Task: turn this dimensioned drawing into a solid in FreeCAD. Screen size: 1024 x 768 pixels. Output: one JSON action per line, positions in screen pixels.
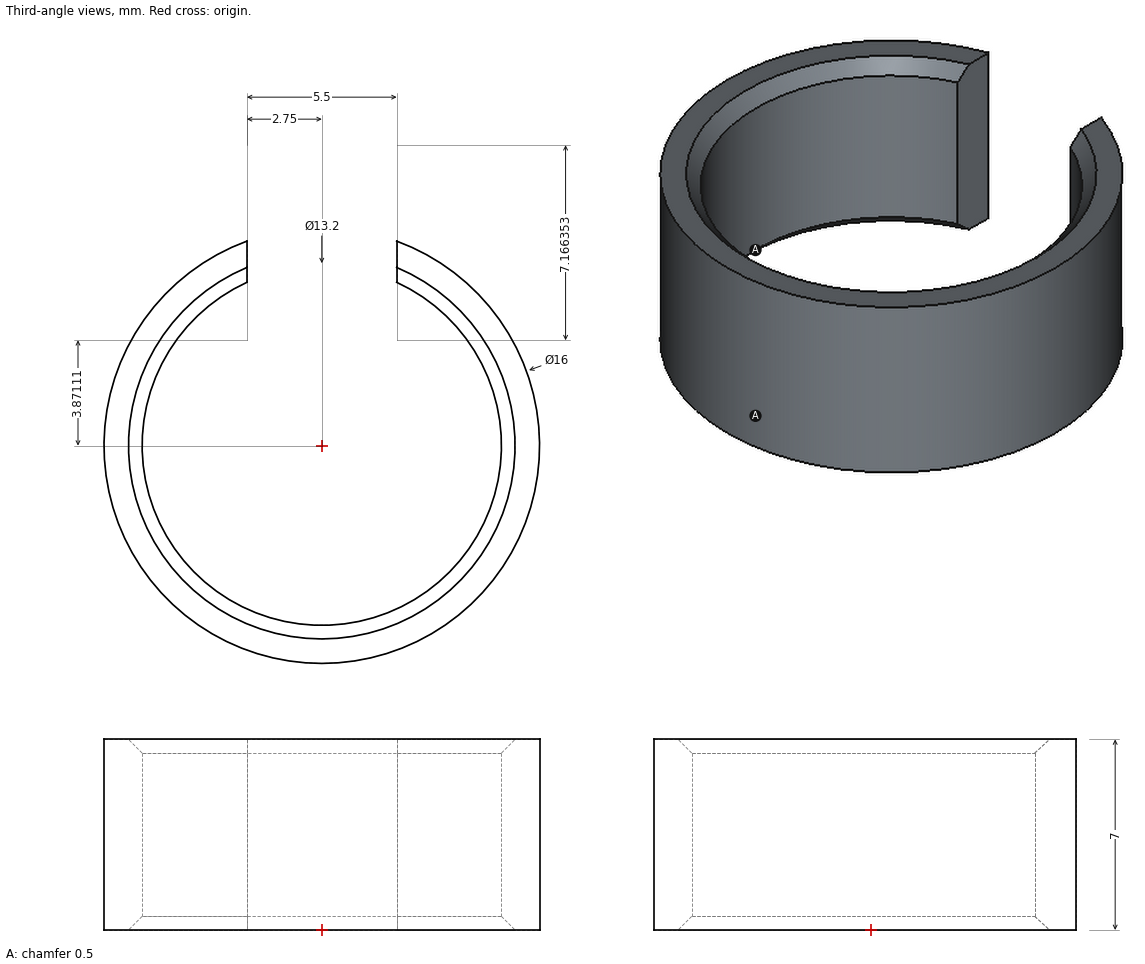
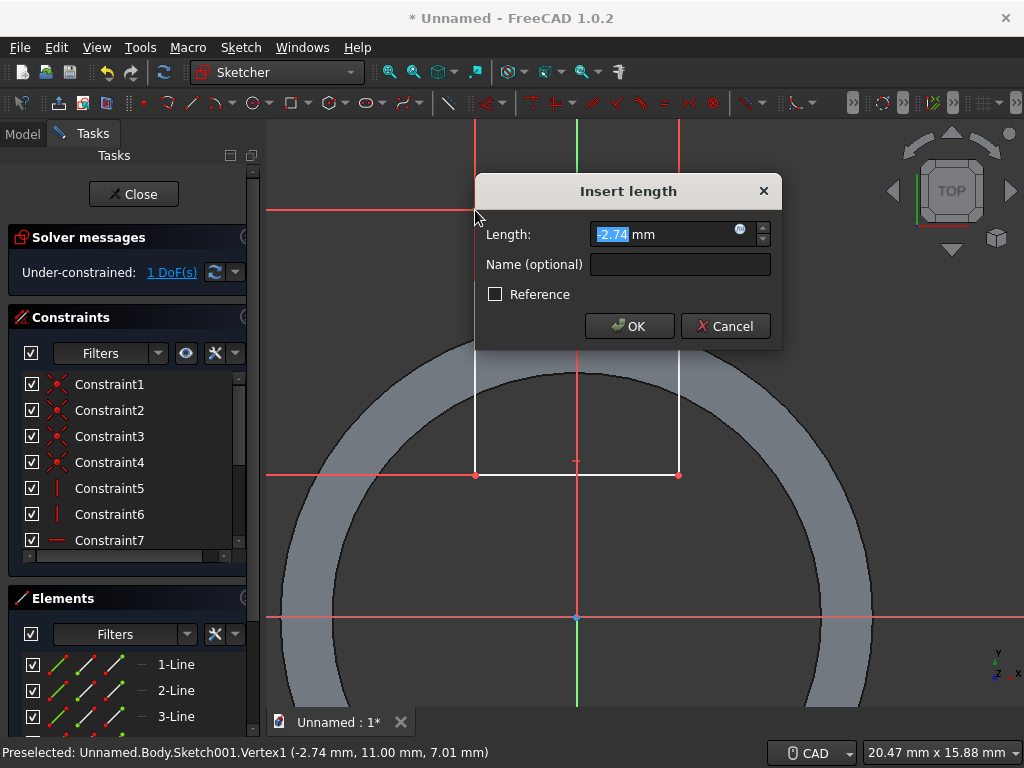
{"action": "type", "text": "-2.75"}
{"action": "key", "text": "Return"}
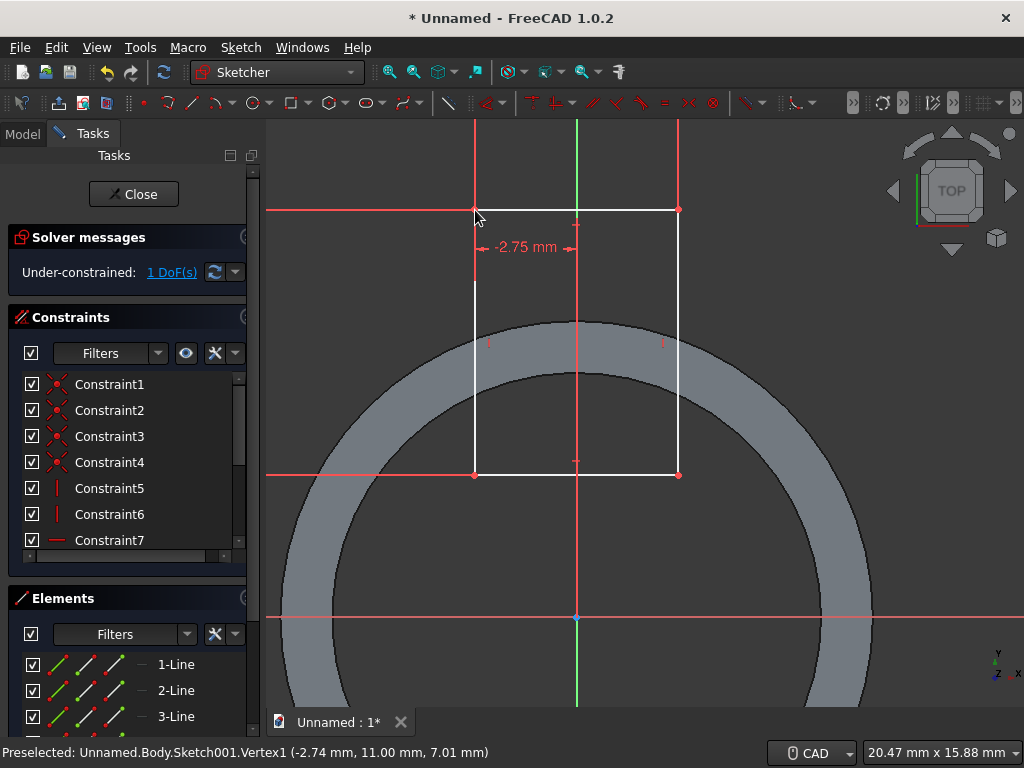
{"action": "left_click", "coordinate": [475, 475]}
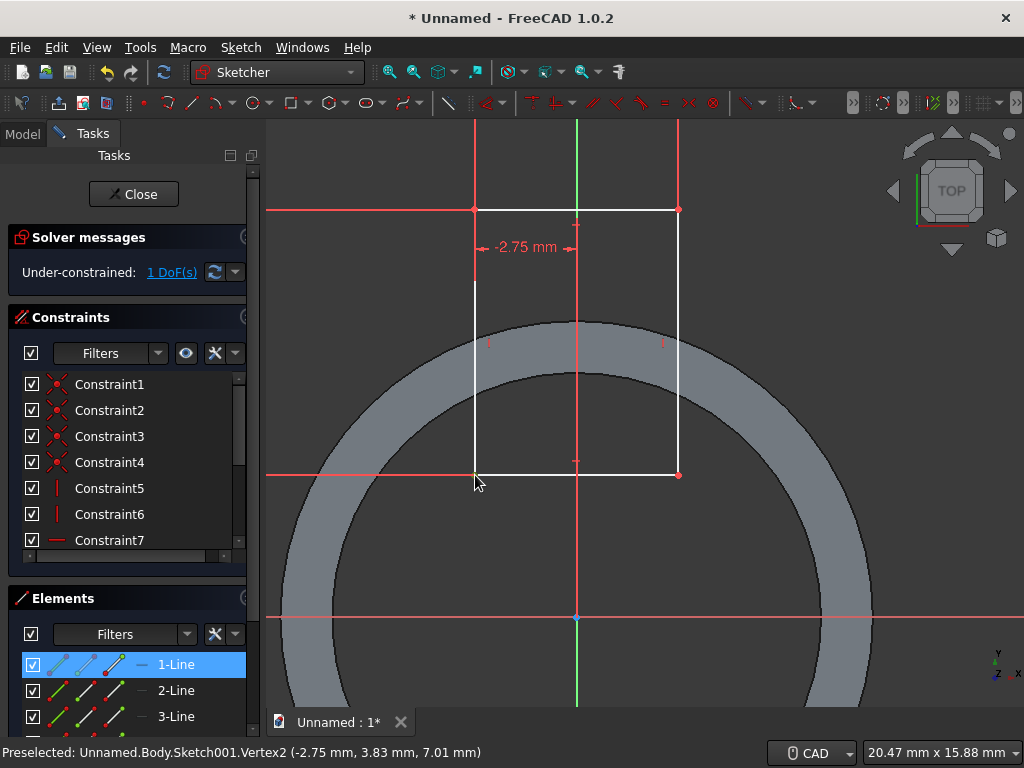
{"action": "key", "text": "i"}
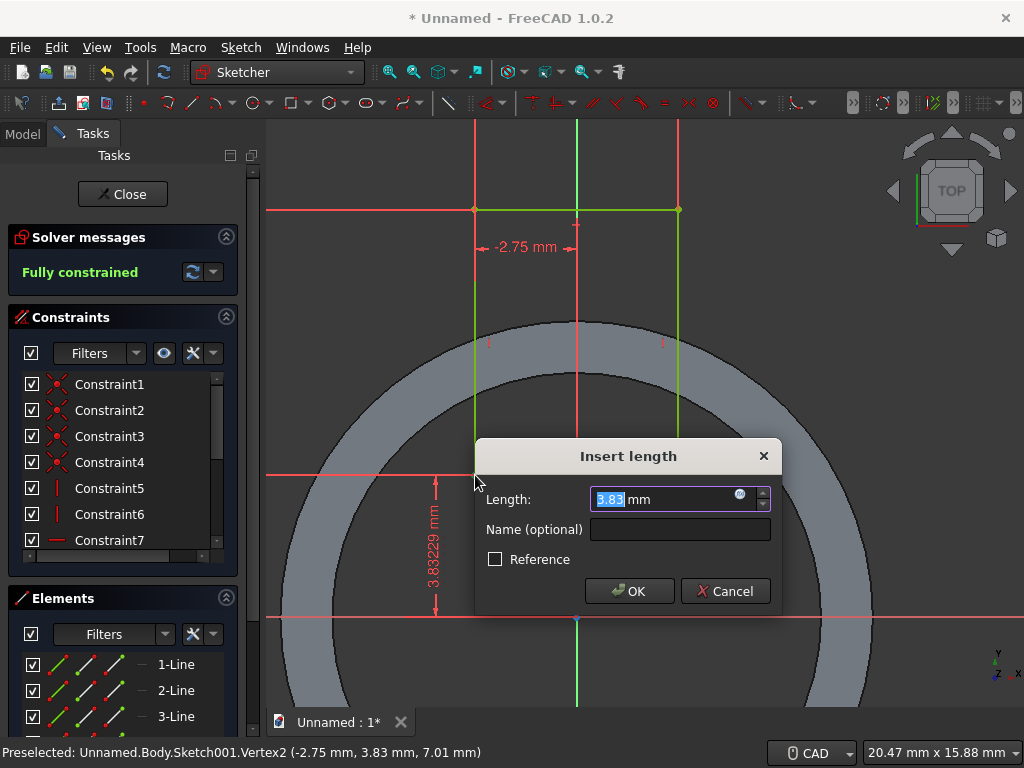
{"action": "type", "text": "3.87111"}
{"action": "key", "text": "Return"}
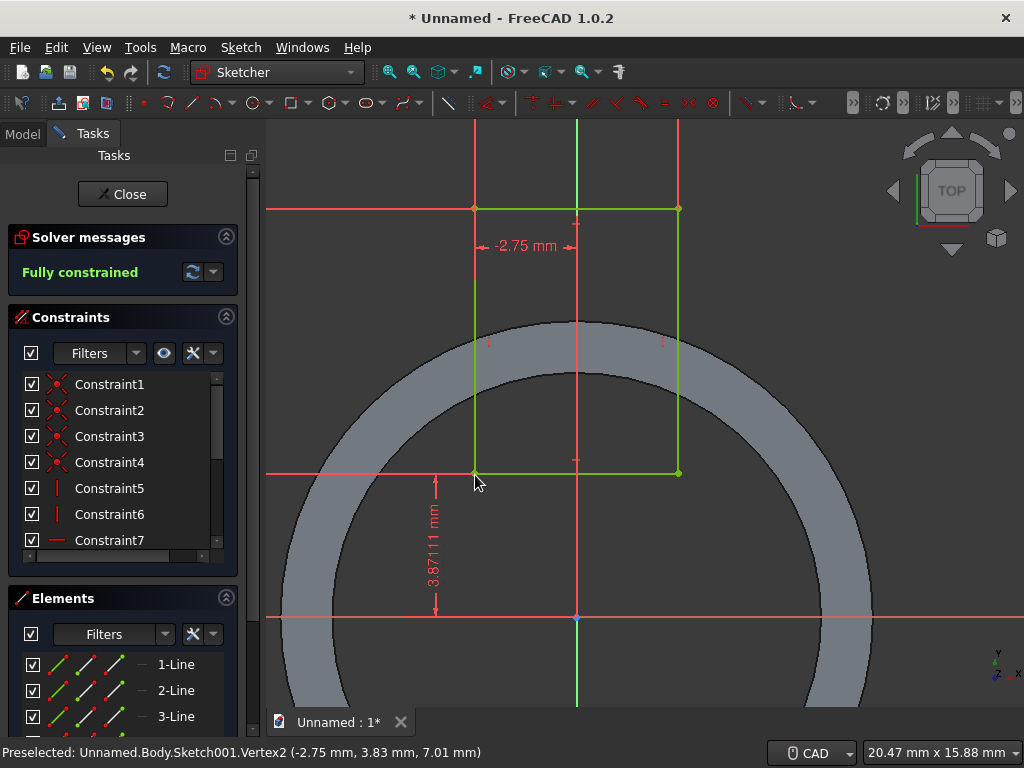
{"action": "left_click", "coordinate": [123, 194]}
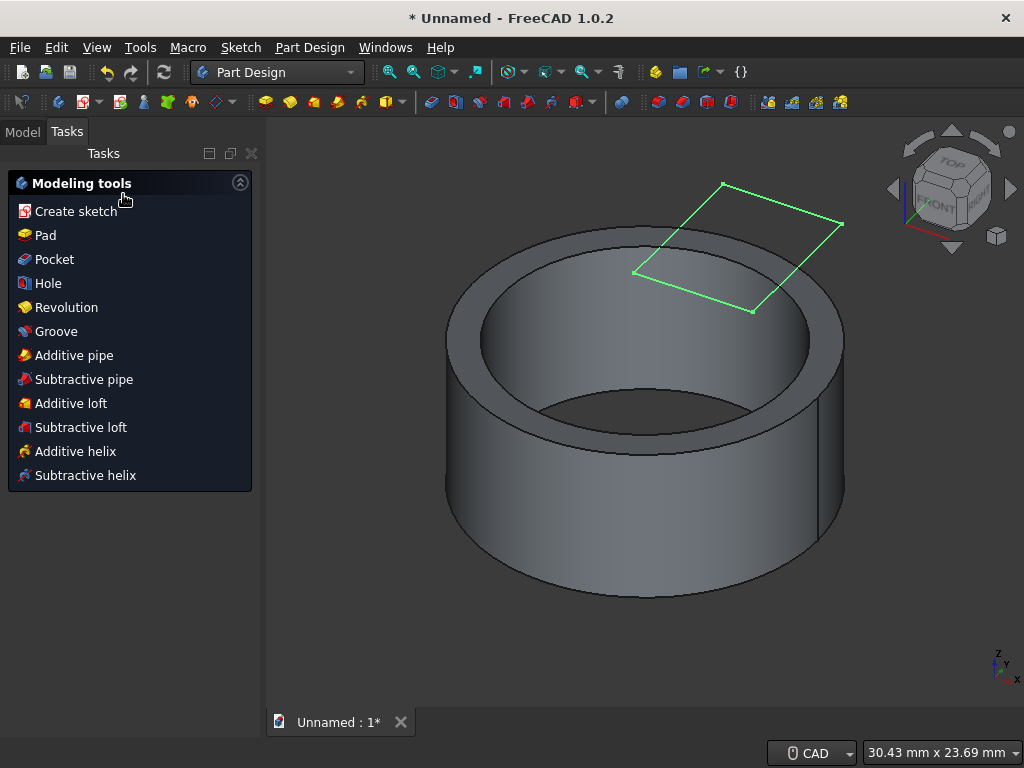
{"action": "left_click", "coordinate": [432, 102]}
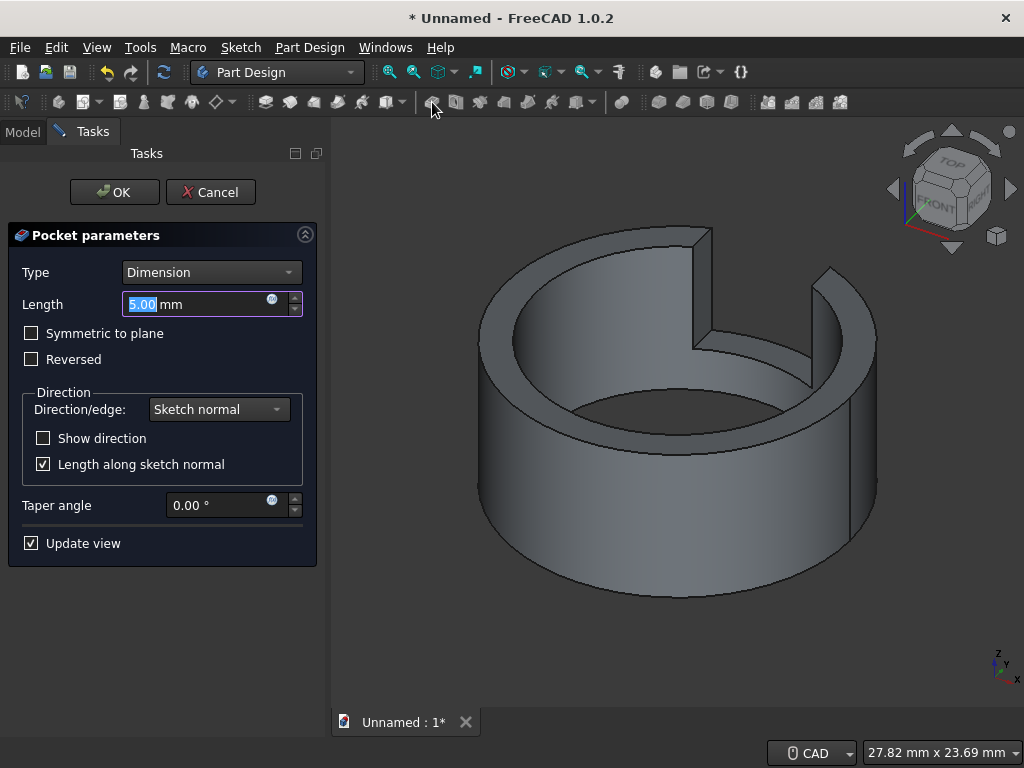
{"action": "left_click", "coordinate": [212, 272]}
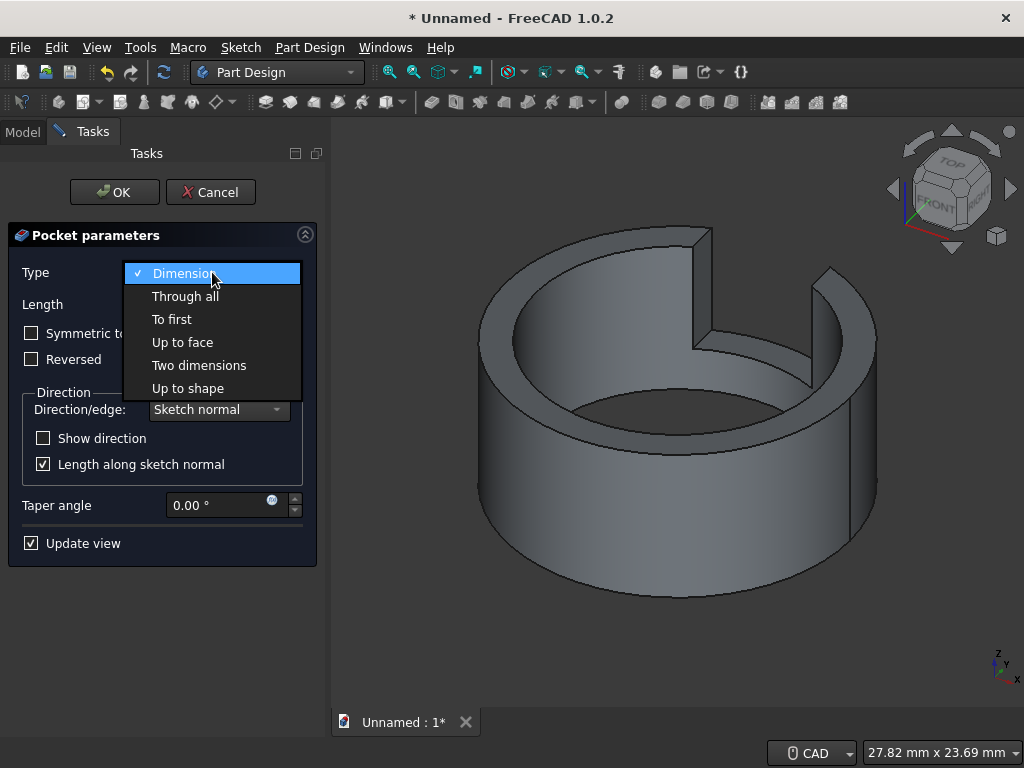
{"action": "left_click", "coordinate": [212, 296]}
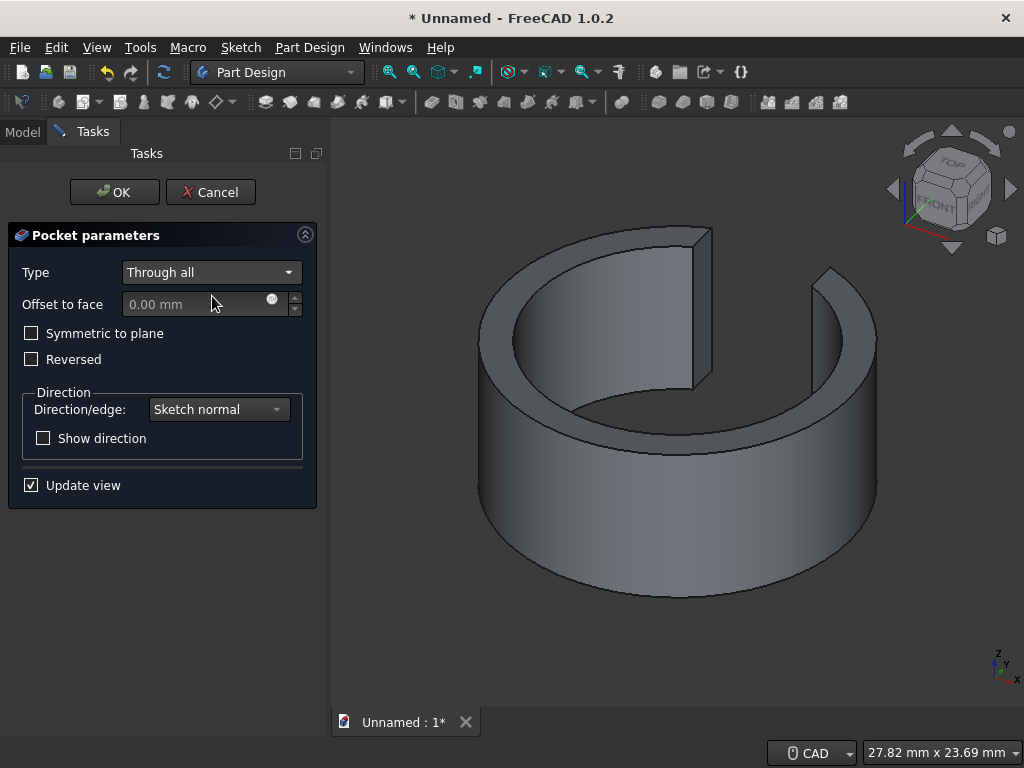
{"action": "left_click", "coordinate": [115, 192]}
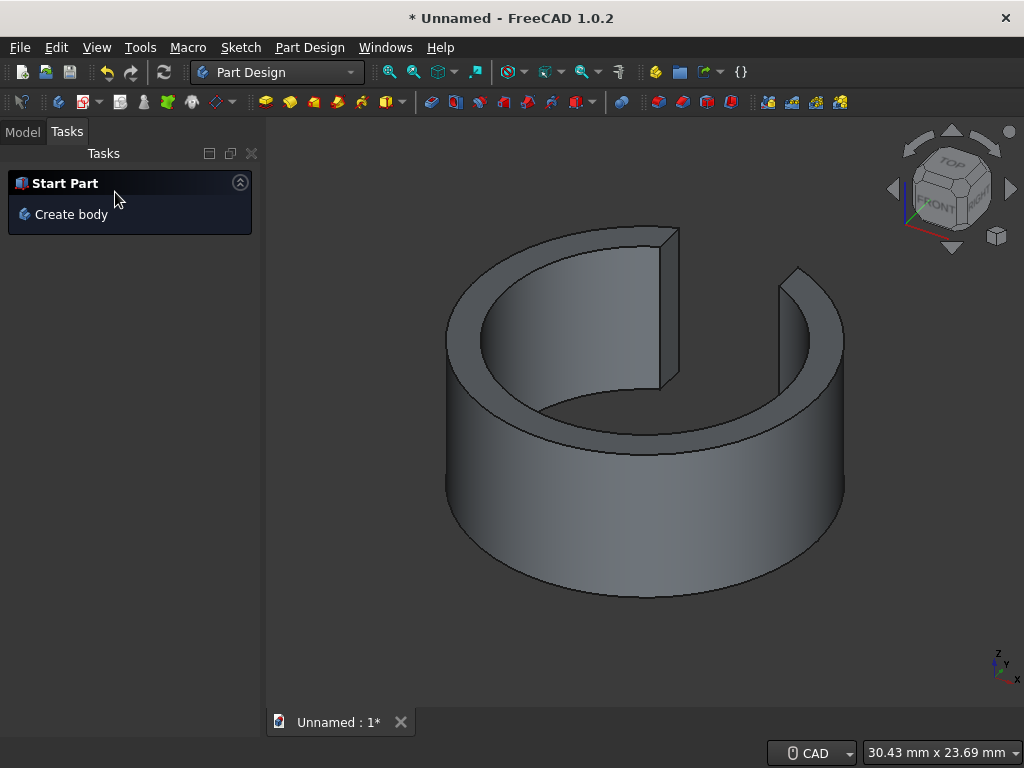
{"action": "left_click", "coordinate": [492, 305]}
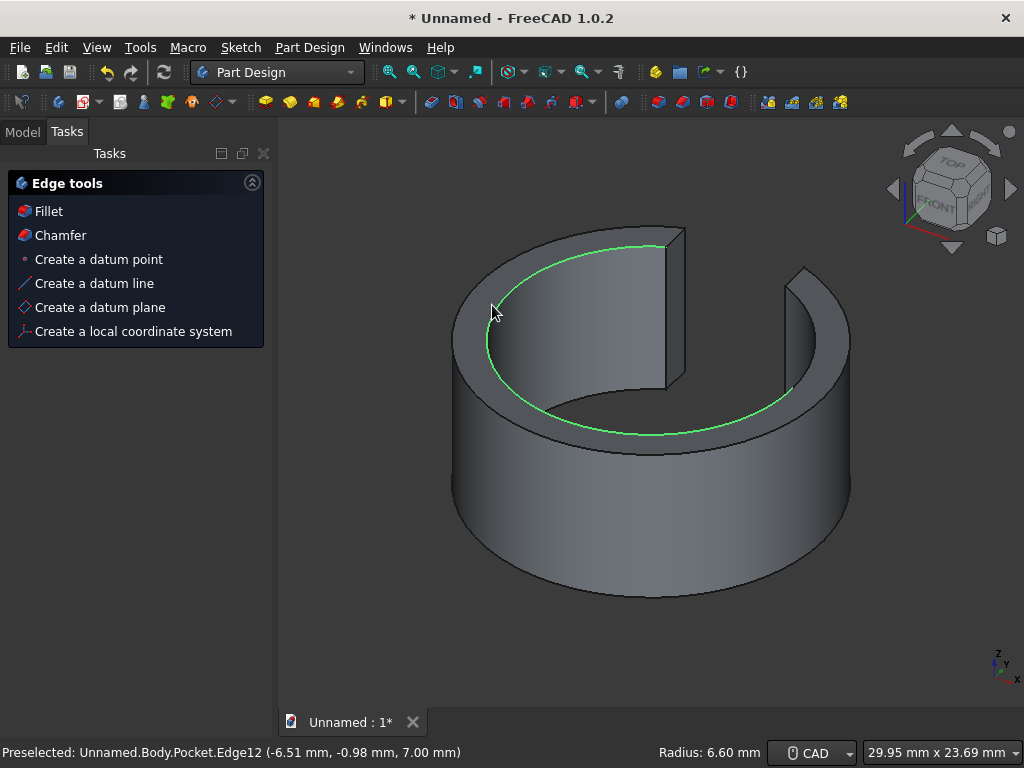
{"action": "key", "text": "0"}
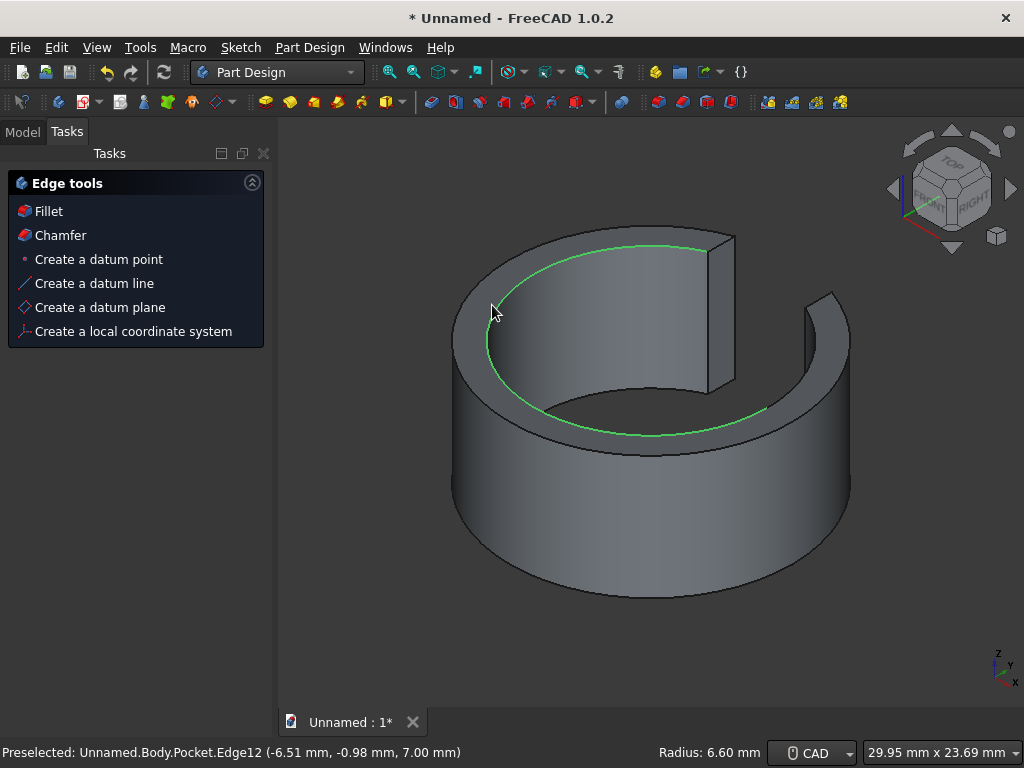
{"action": "key", "text": "2"}